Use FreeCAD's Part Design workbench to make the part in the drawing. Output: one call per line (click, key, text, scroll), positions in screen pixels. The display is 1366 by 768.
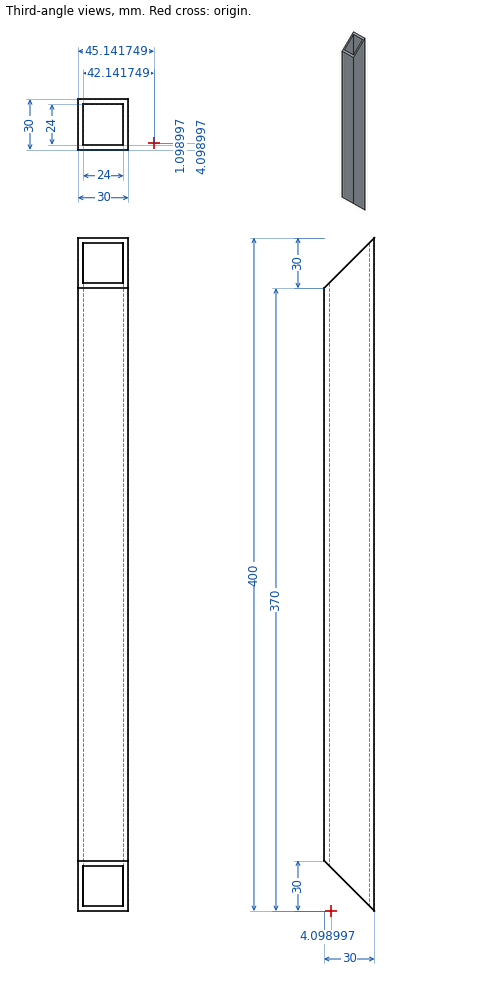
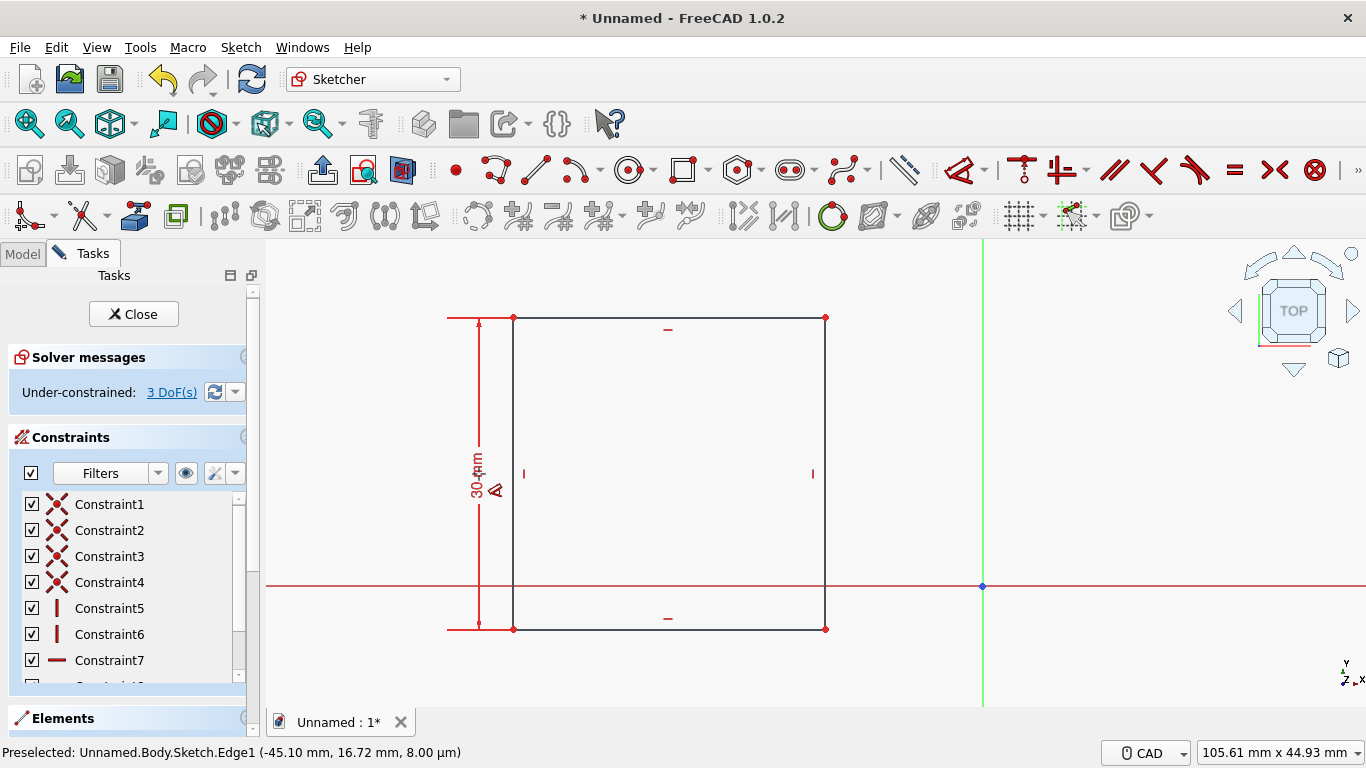
click(607, 630)
click(669, 664)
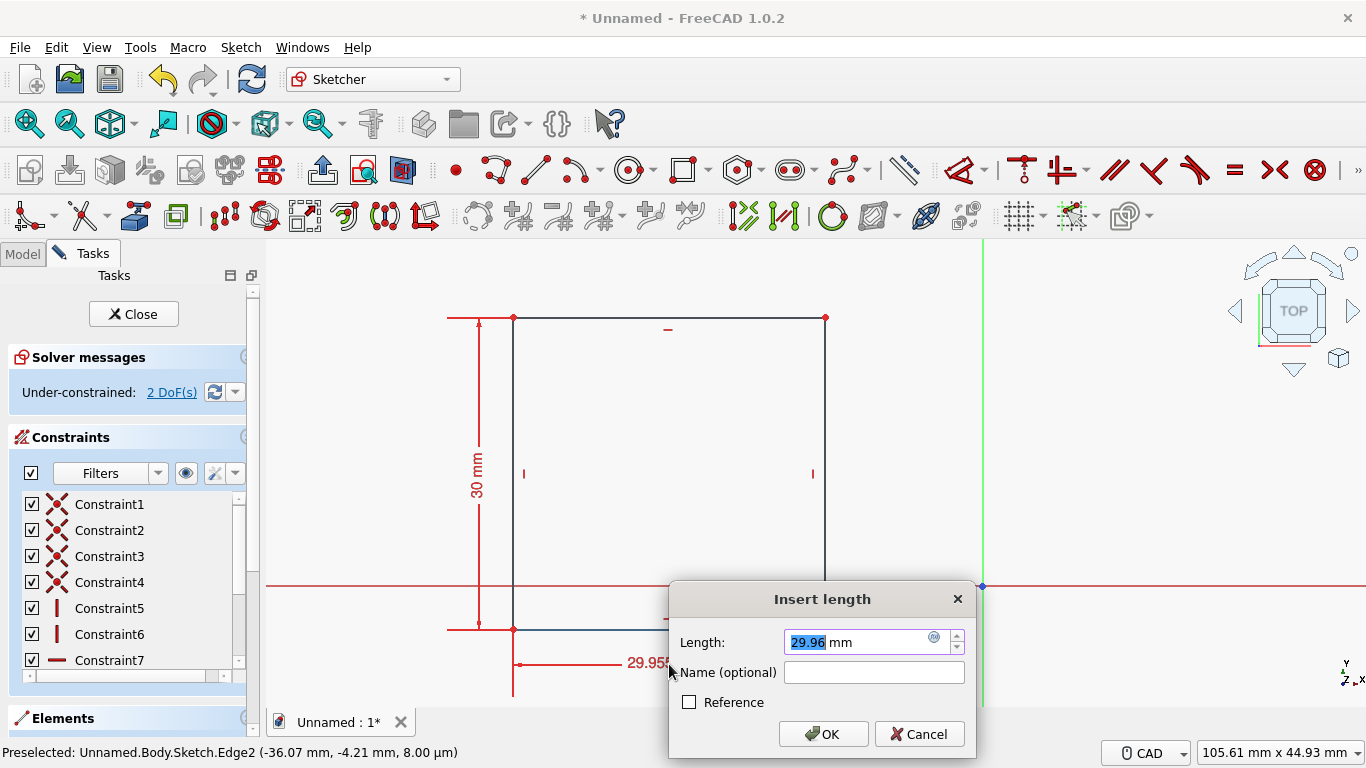
text(30)
key(Return)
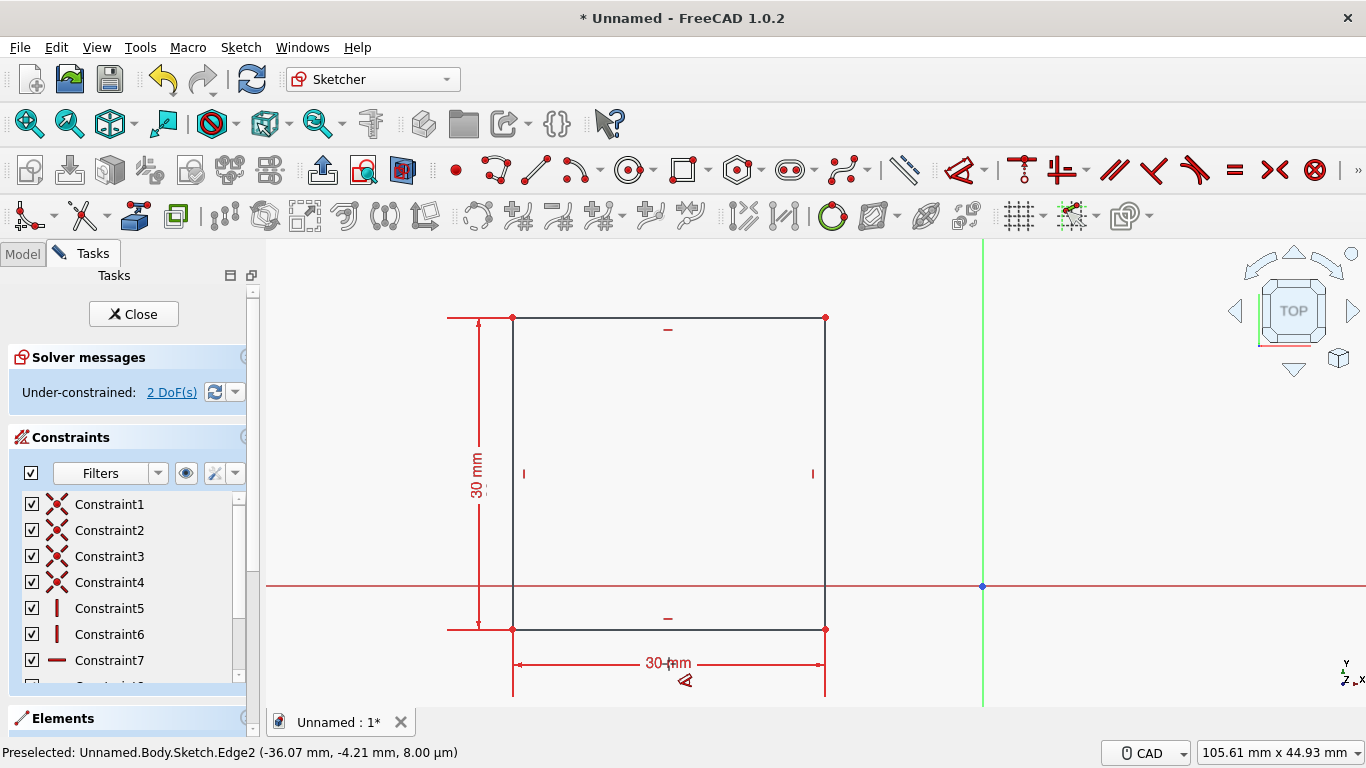
click(513, 630)
click(479, 608)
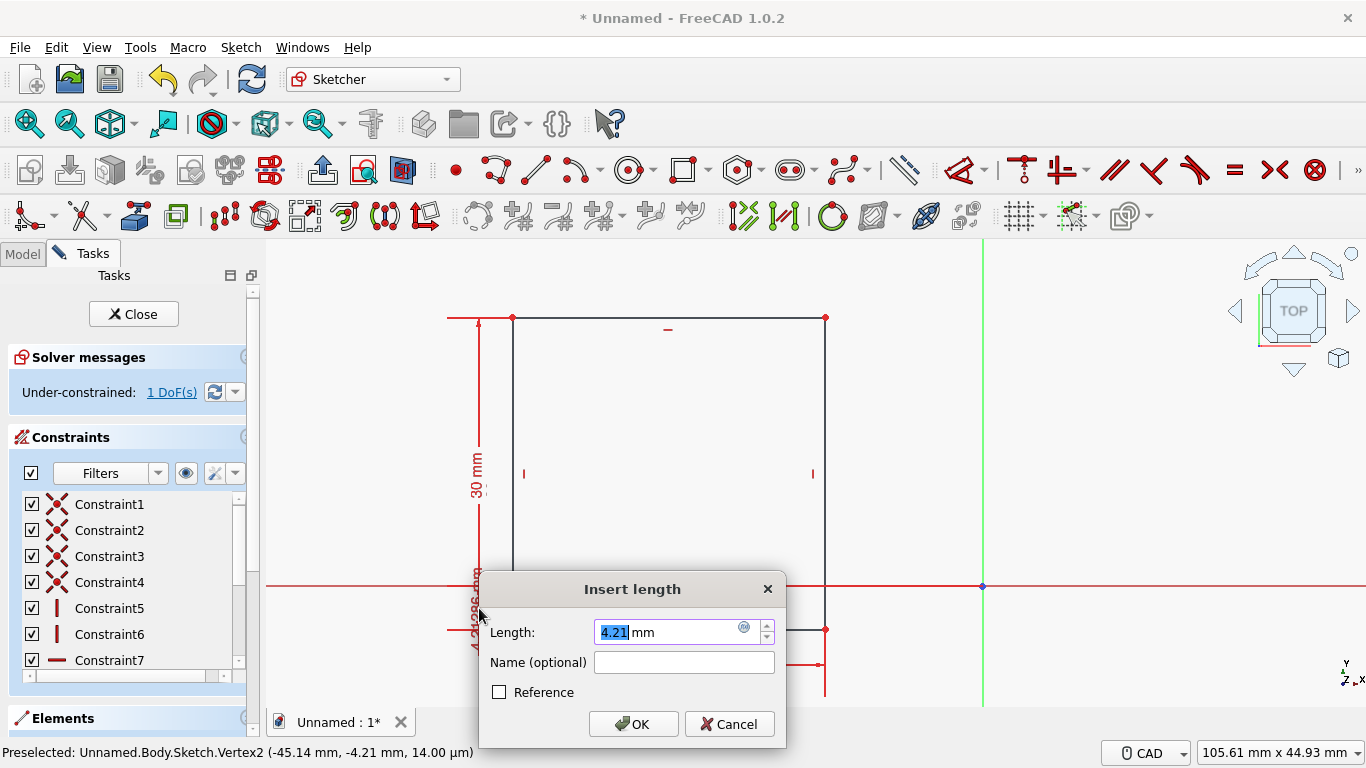
text(4.098997)
key(Return)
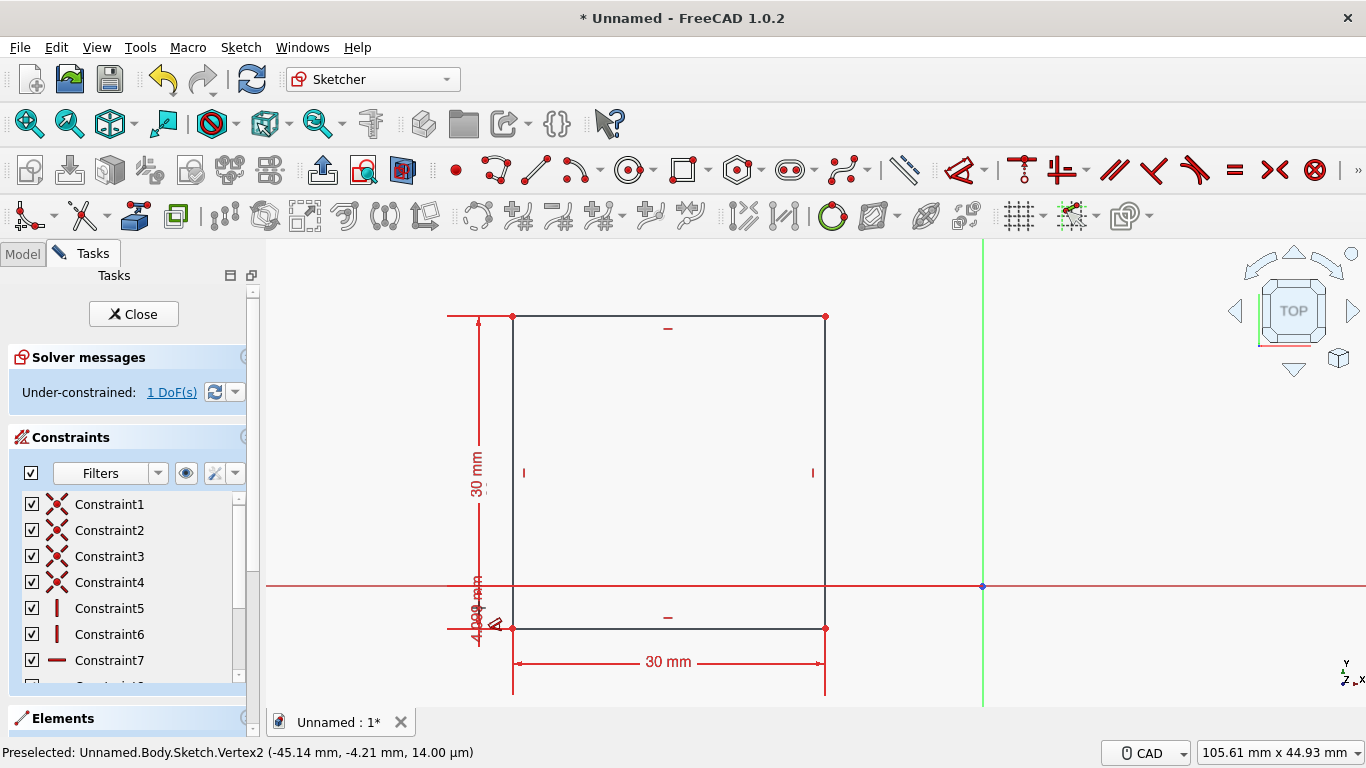
click(513, 316)
click(748, 282)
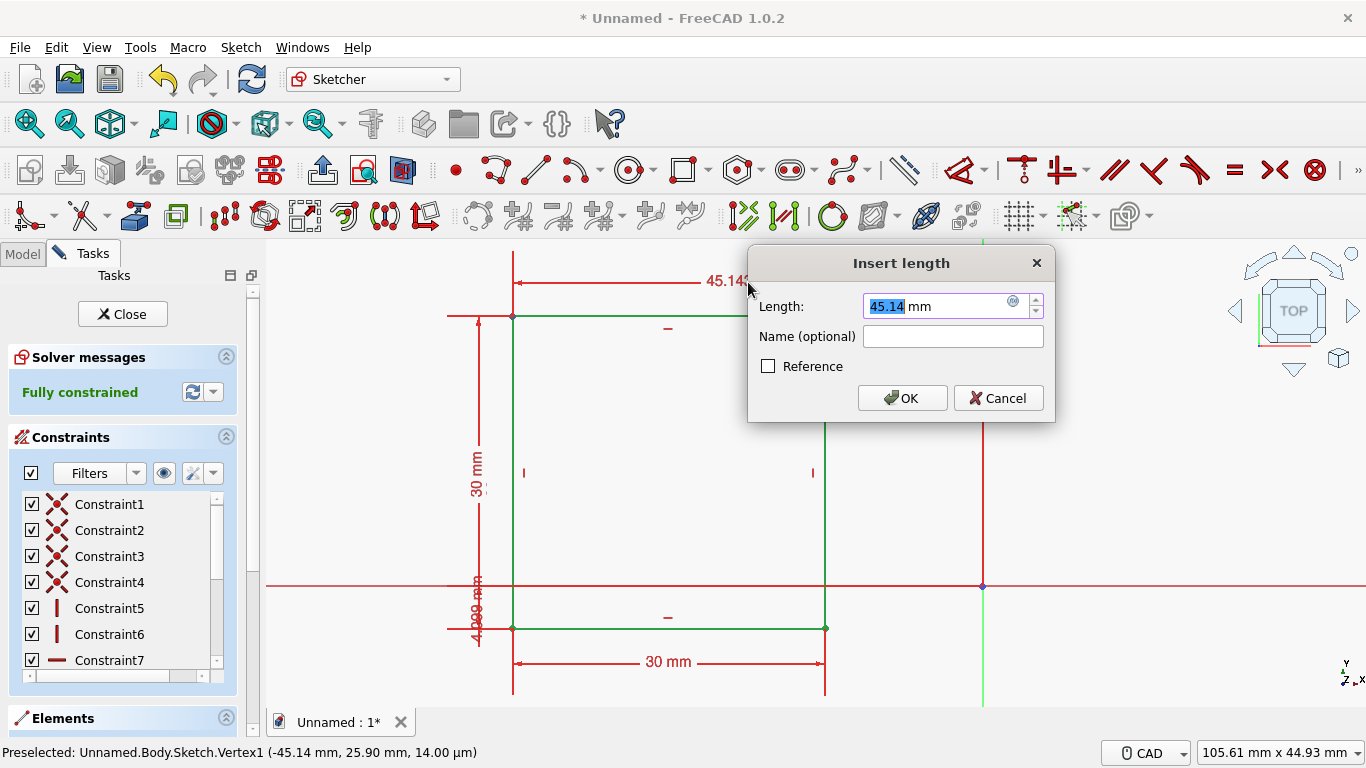
text(45.141749)
key(Return)
key(Escape)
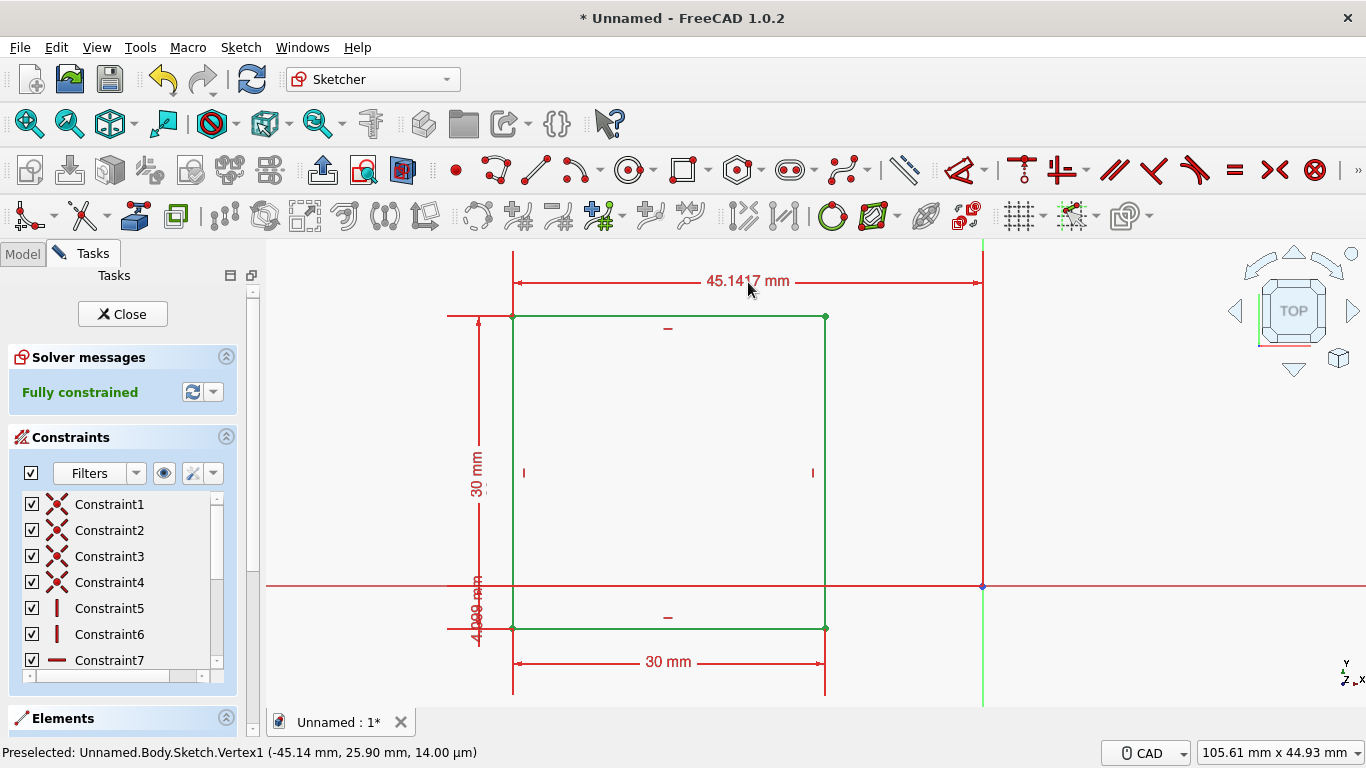
click(123, 314)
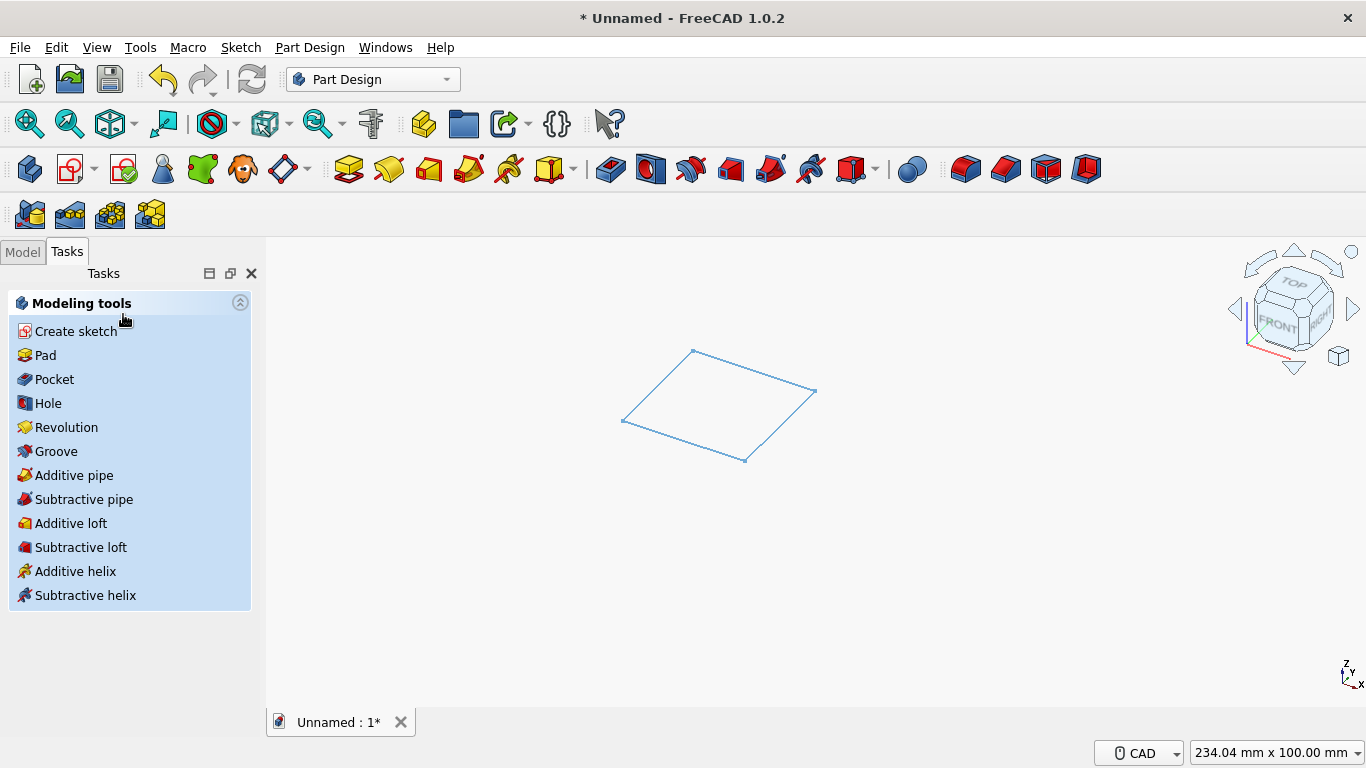
click(350, 170)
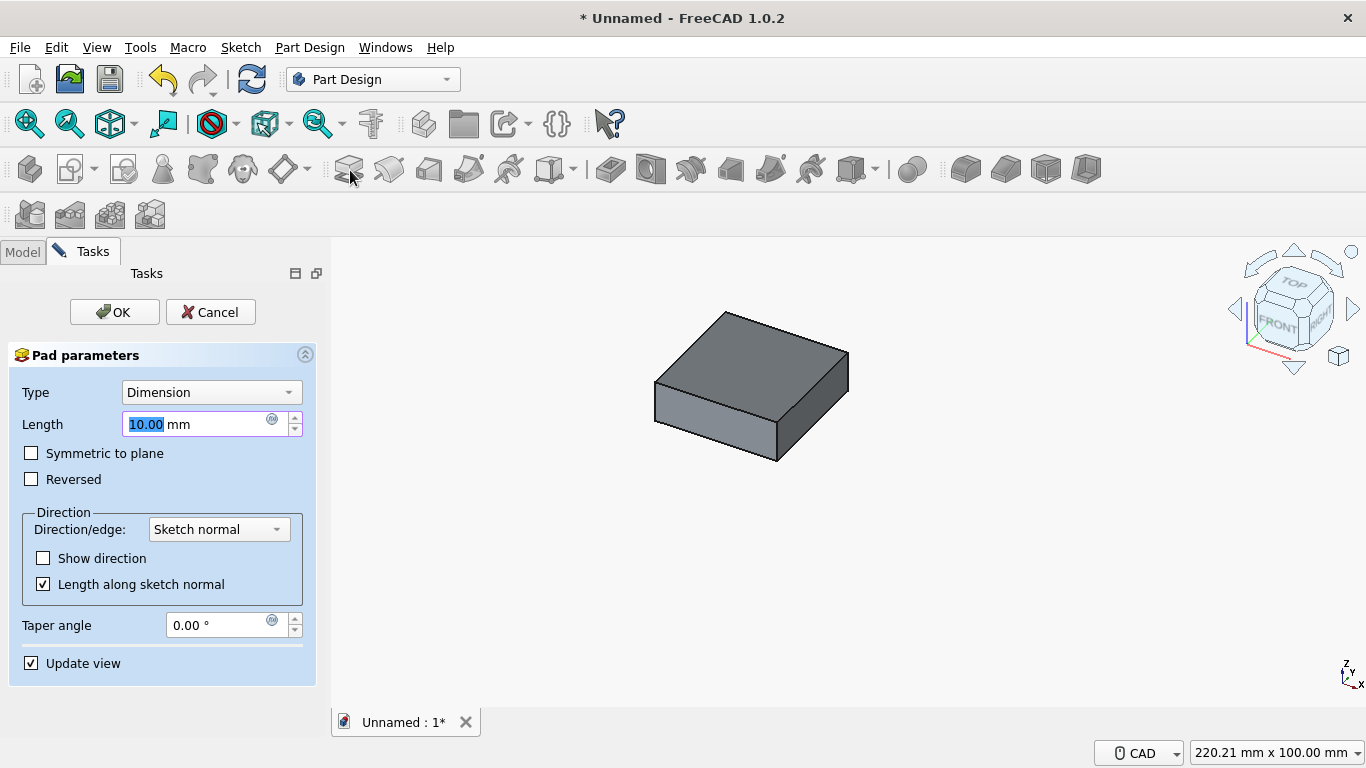
text(400)
key(Tab)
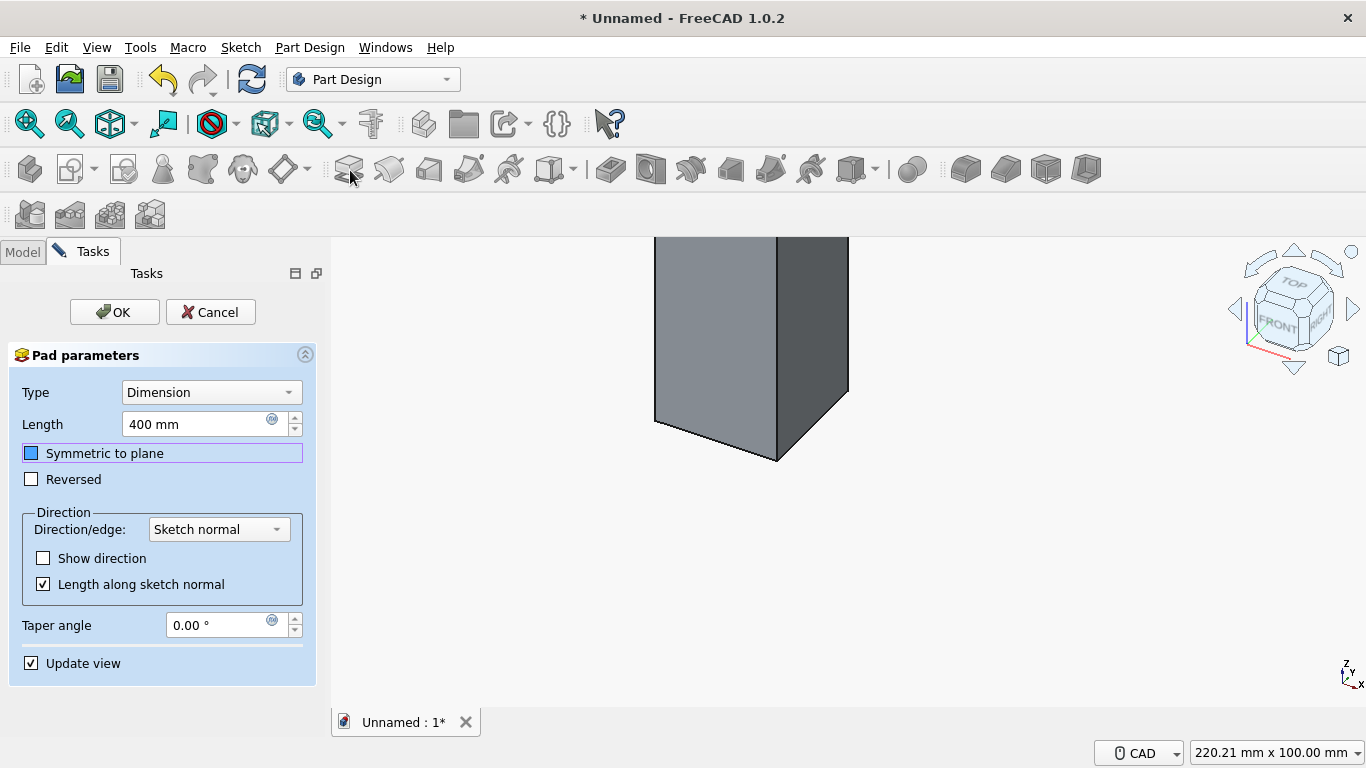
click(115, 312)